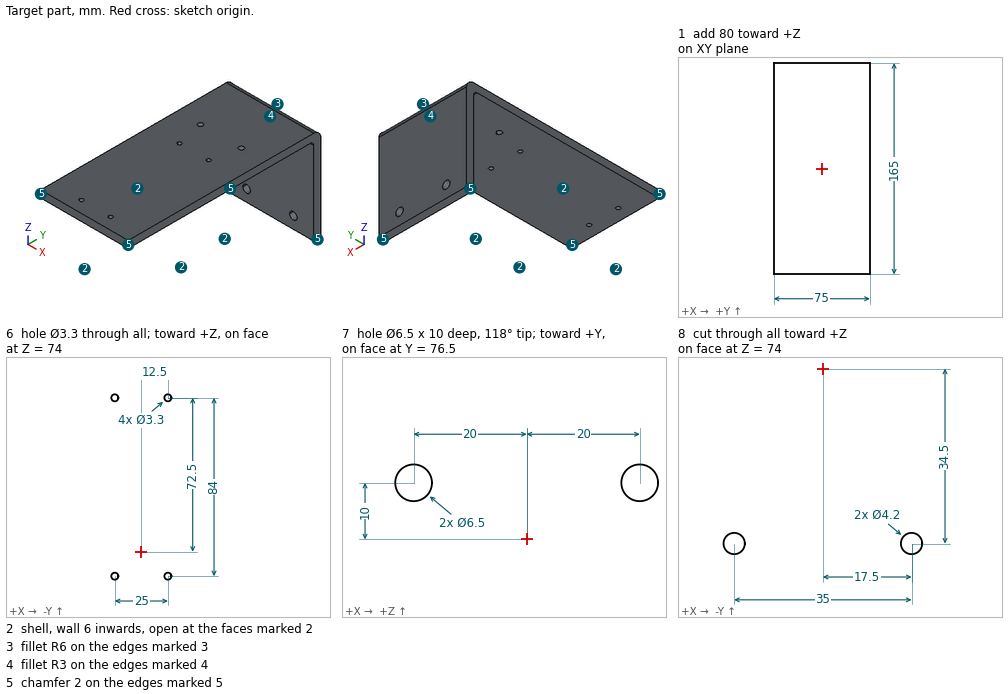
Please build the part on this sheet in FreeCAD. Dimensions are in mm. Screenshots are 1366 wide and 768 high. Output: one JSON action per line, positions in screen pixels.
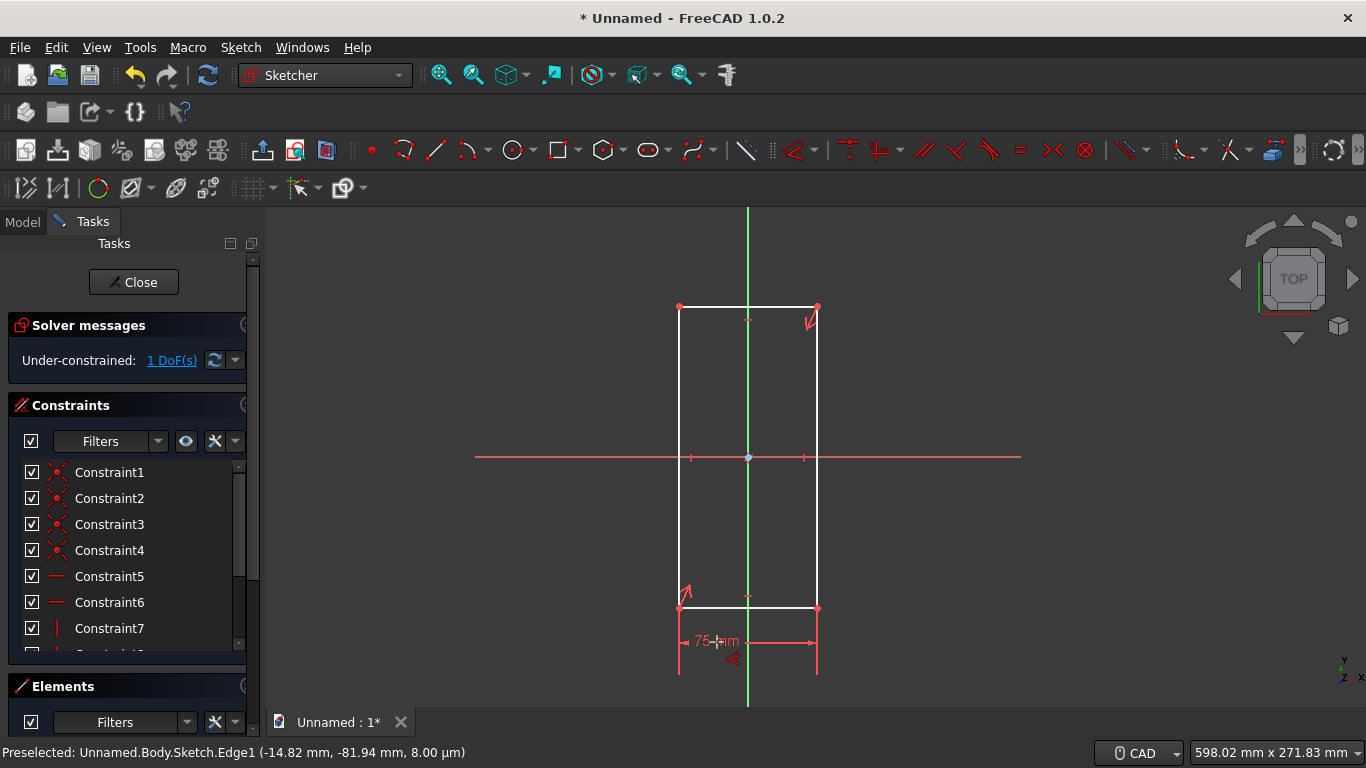
{"action": "left_click", "coordinate": [817, 518]}
{"action": "left_click", "coordinate": [851, 388]}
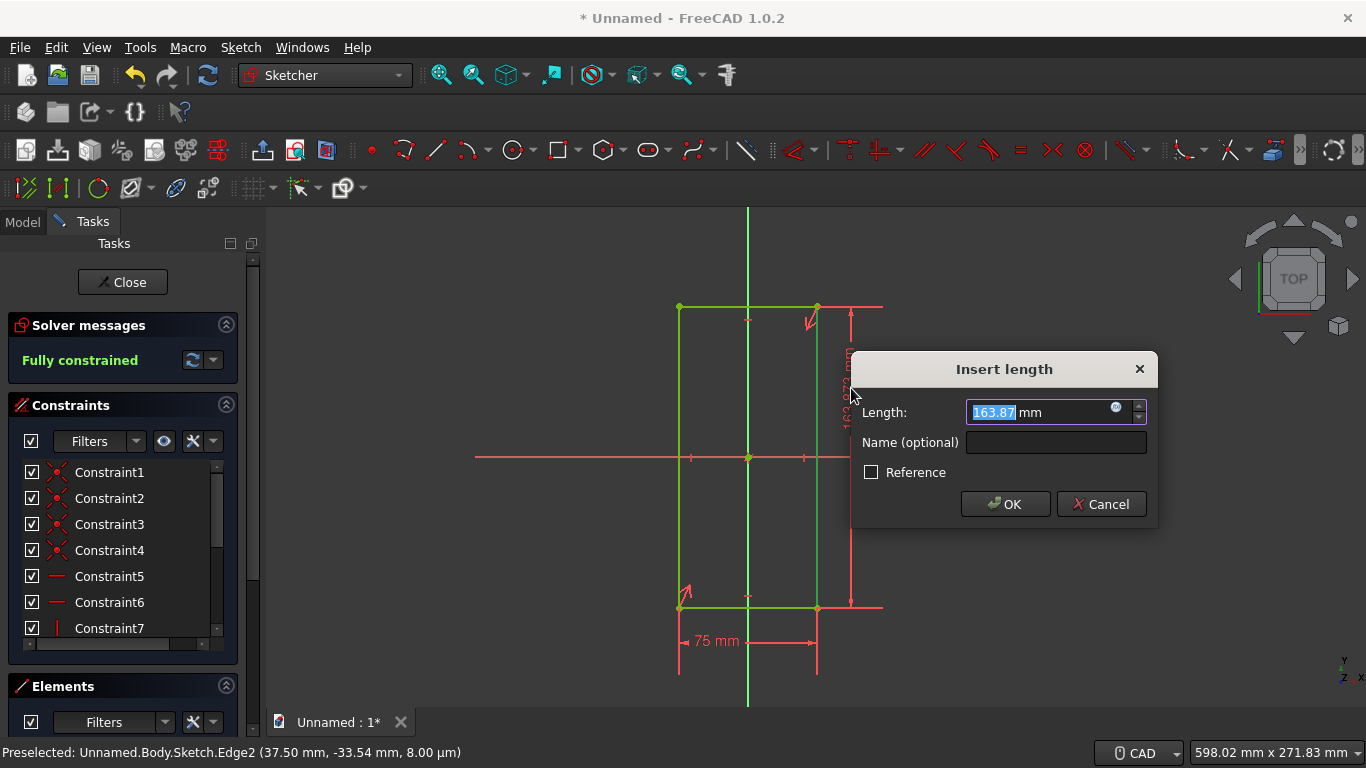
{"action": "type", "text": "165"}
{"action": "key", "text": "Return"}
{"action": "key", "text": "Escape"}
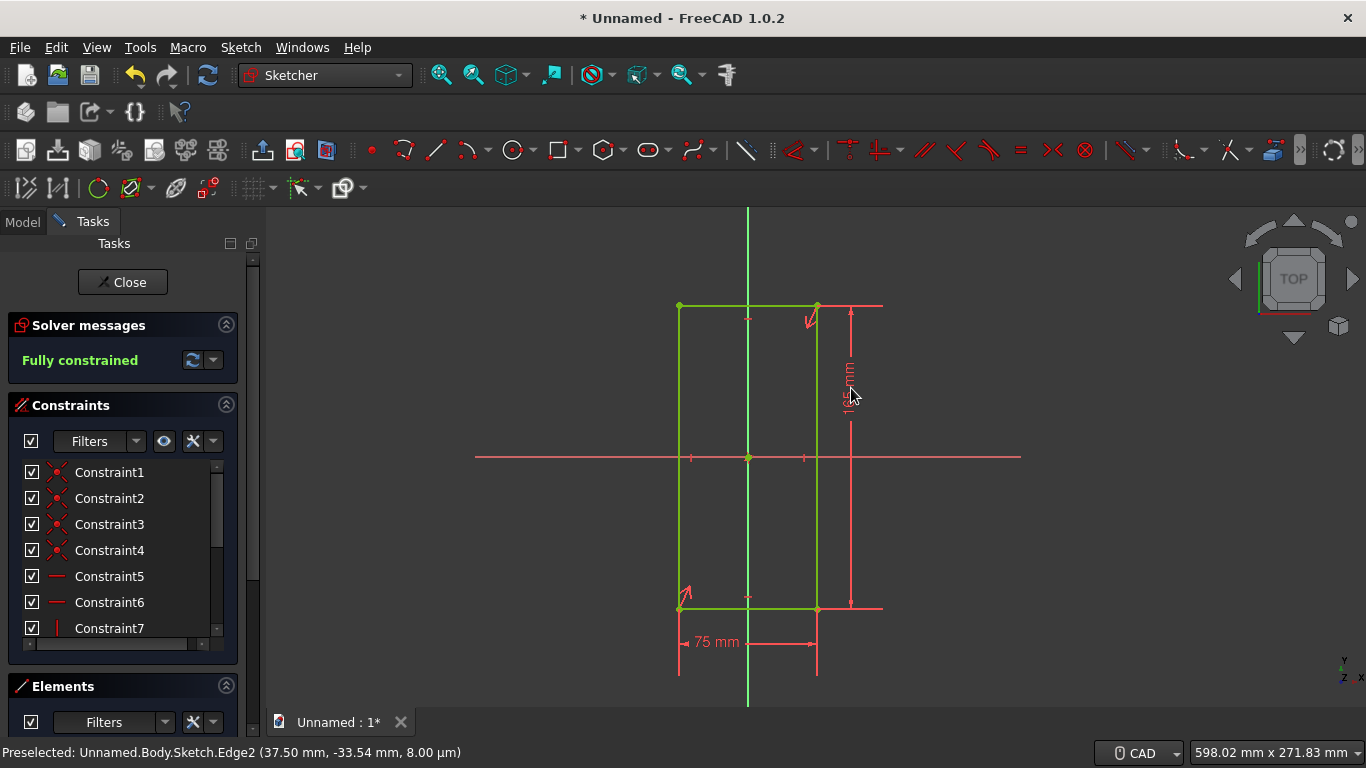
{"action": "left_click", "coordinate": [123, 282]}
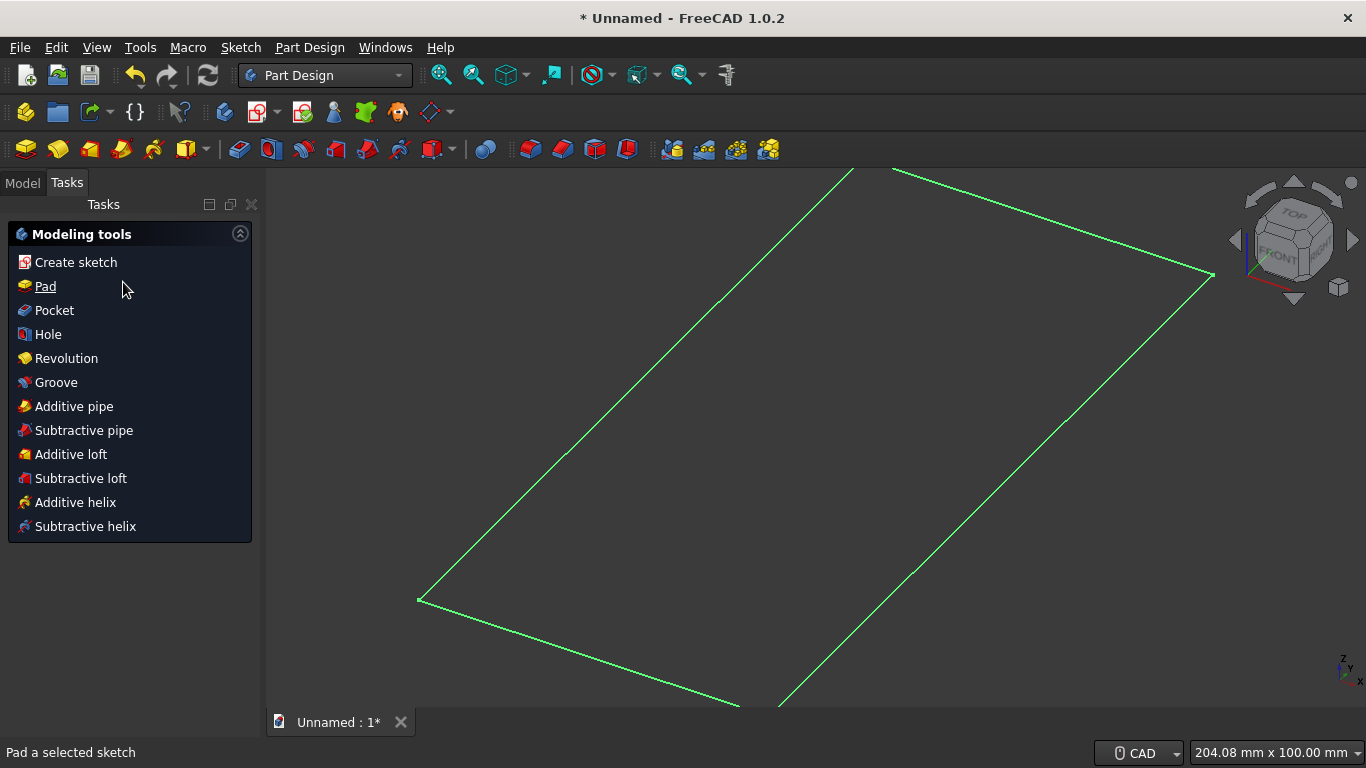
{"action": "left_click", "coordinate": [26, 150]}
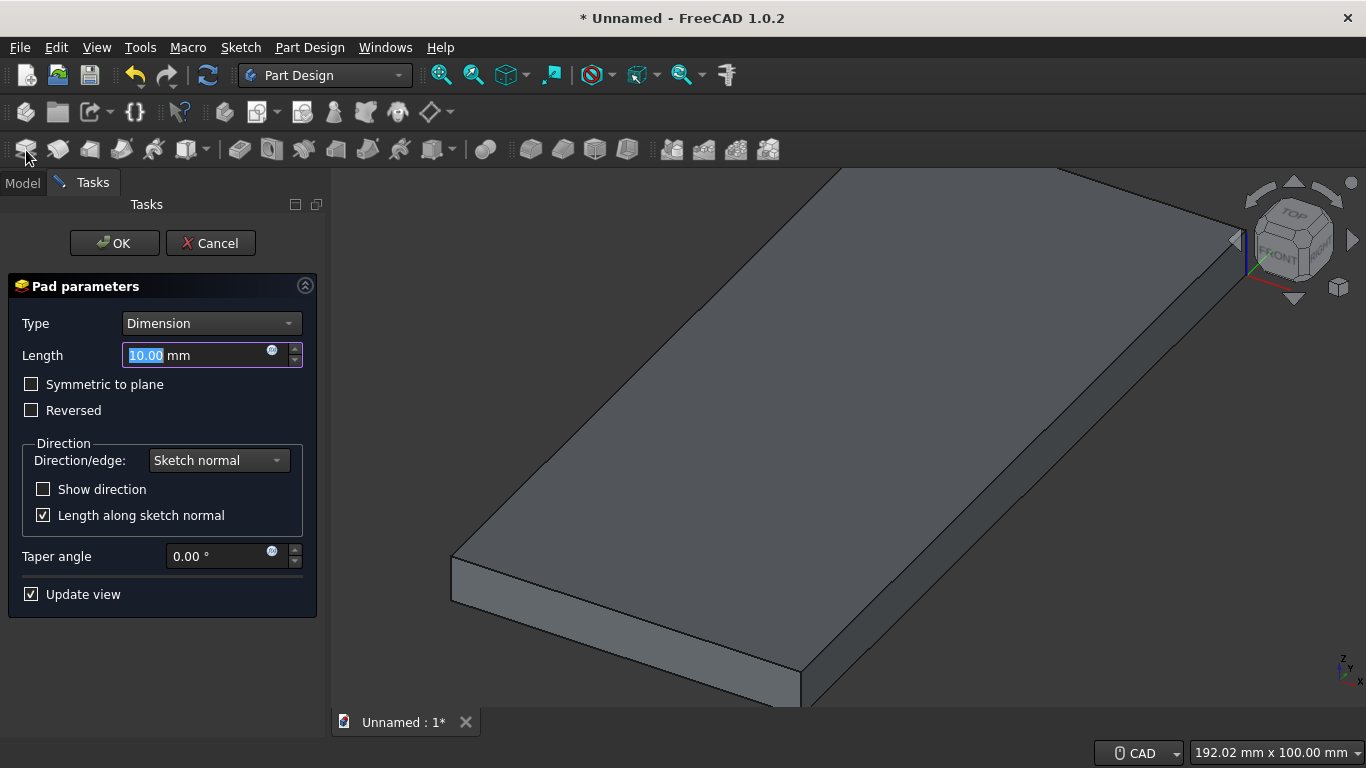
{"action": "type", "text": "80"}
{"action": "key", "text": "Tab"}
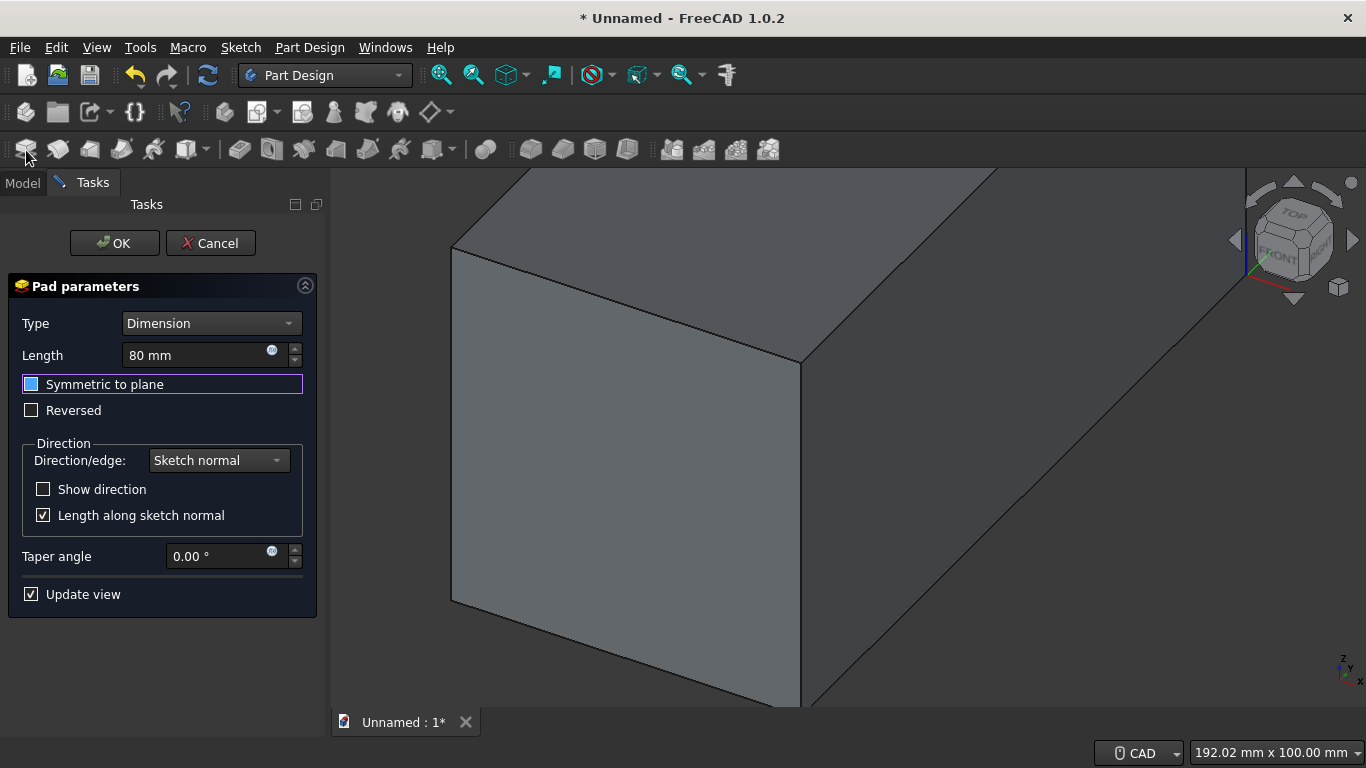
{"action": "left_click", "coordinate": [115, 243]}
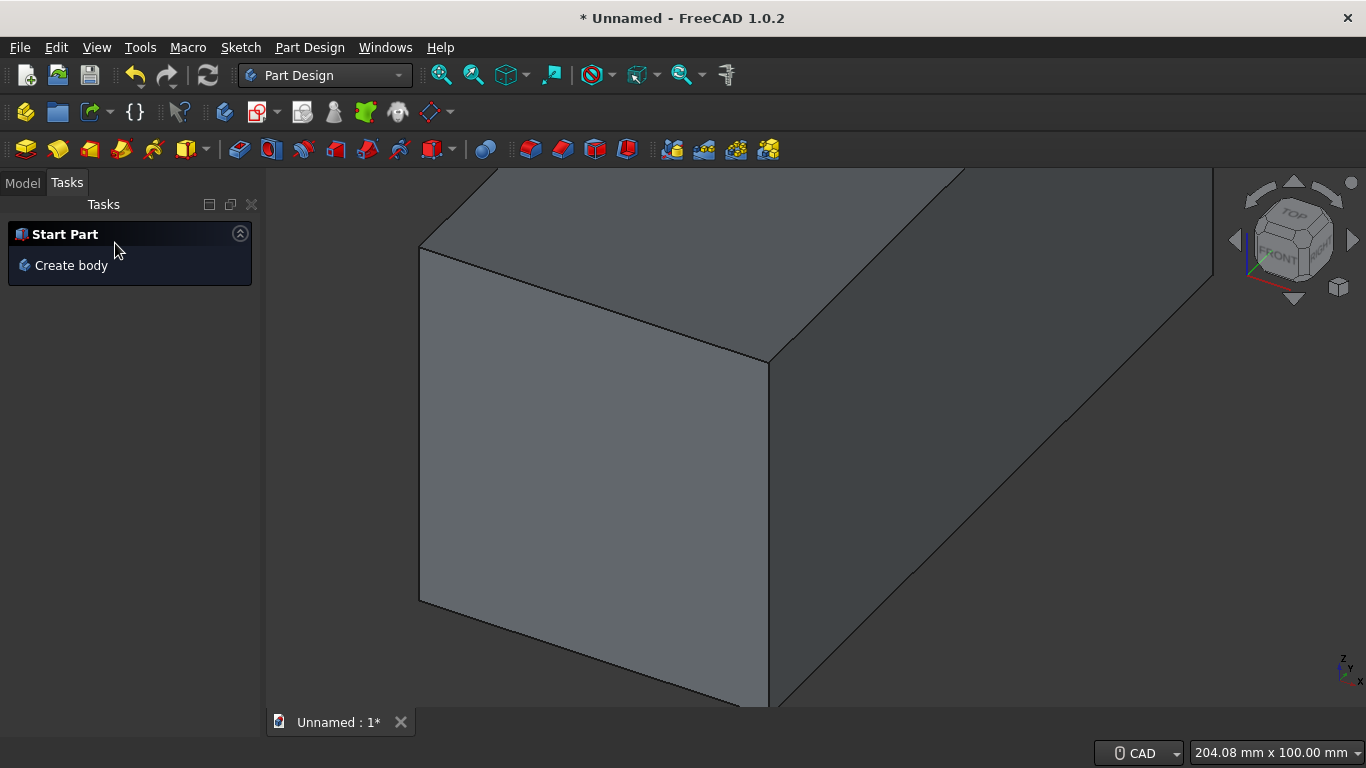
{"action": "left_click", "coordinate": [442, 76]}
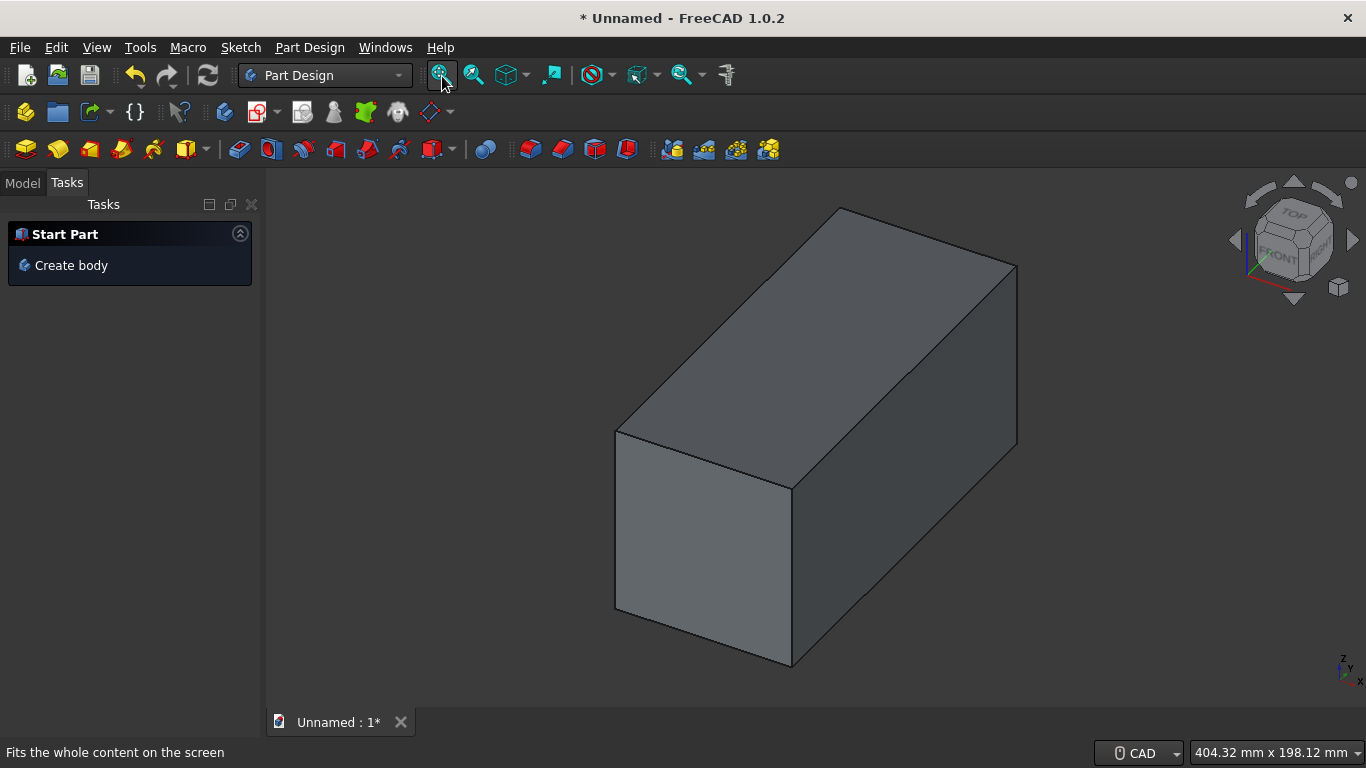
{"action": "left_click", "coordinate": [704, 548]}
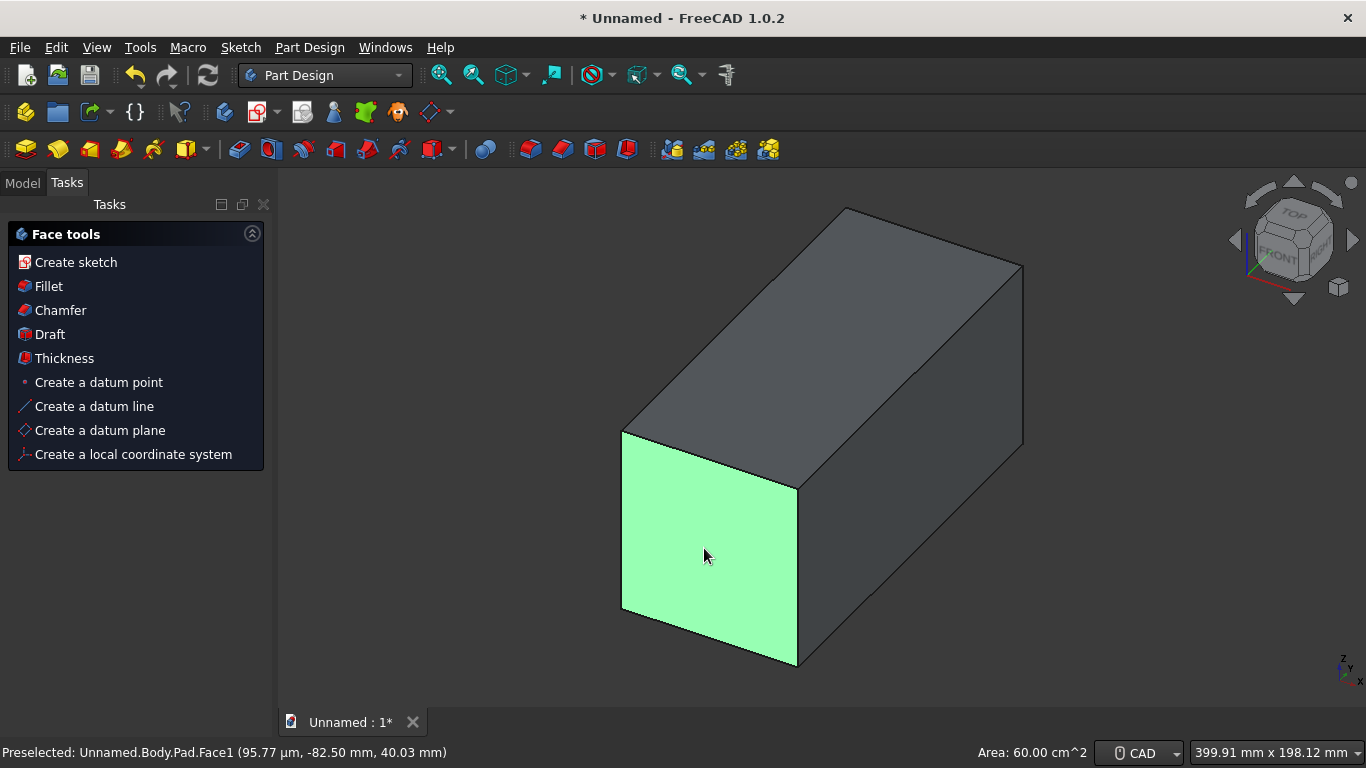
{"action": "left_click", "coordinate": [942, 434], "text": "ctrl"}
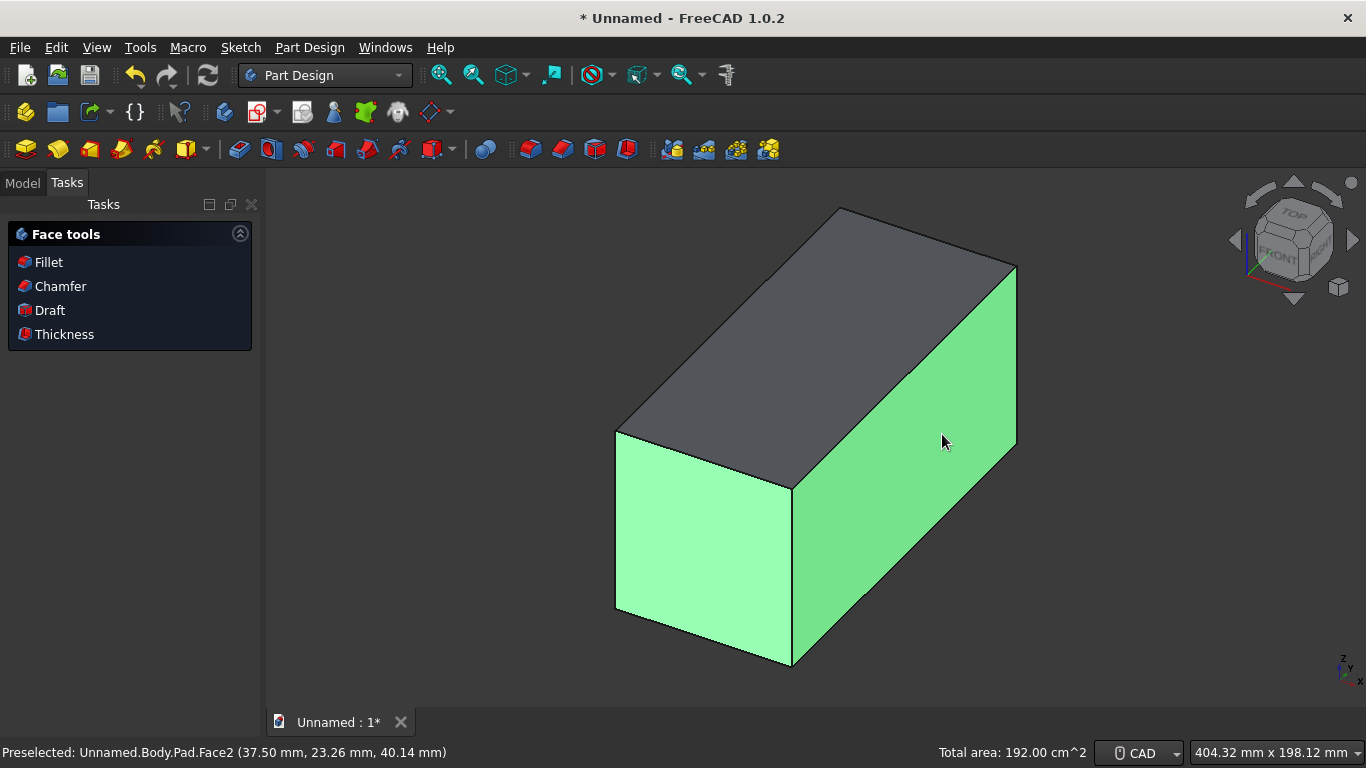
{"action": "key", "text": "0"}